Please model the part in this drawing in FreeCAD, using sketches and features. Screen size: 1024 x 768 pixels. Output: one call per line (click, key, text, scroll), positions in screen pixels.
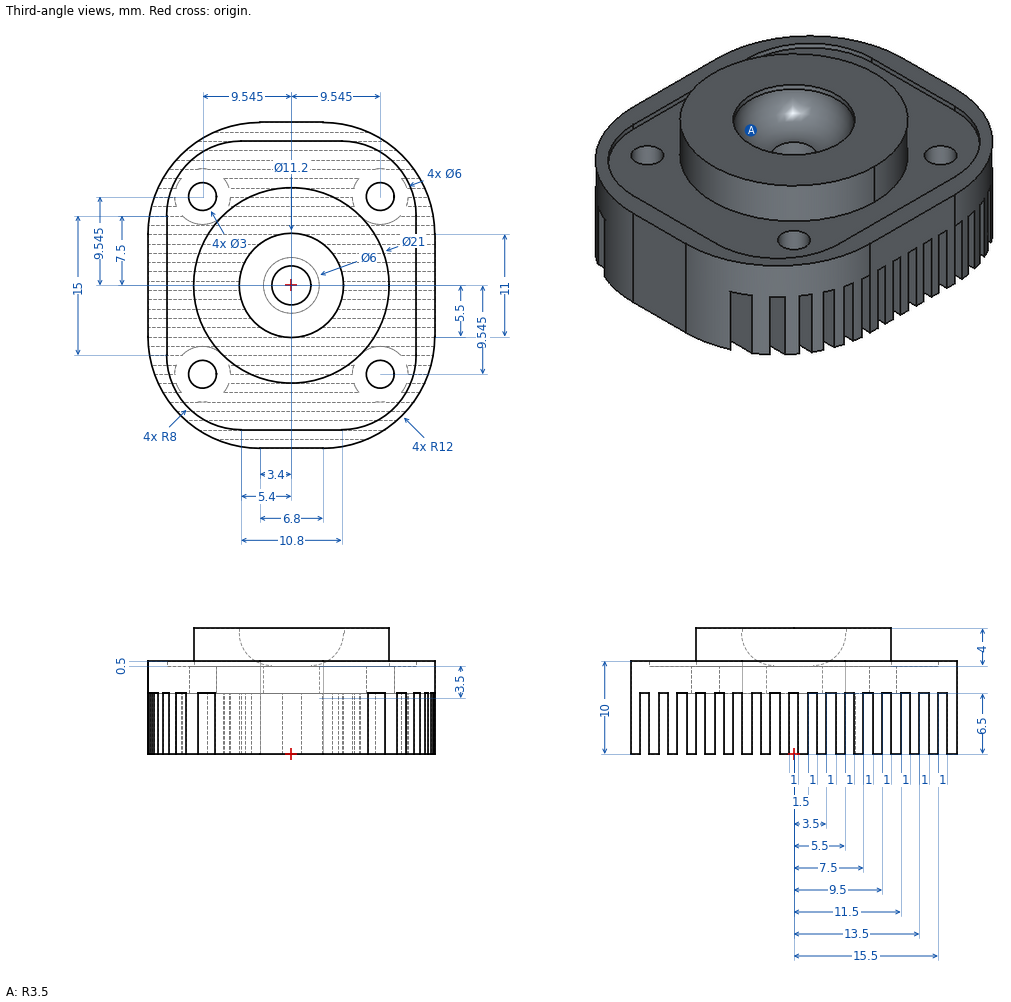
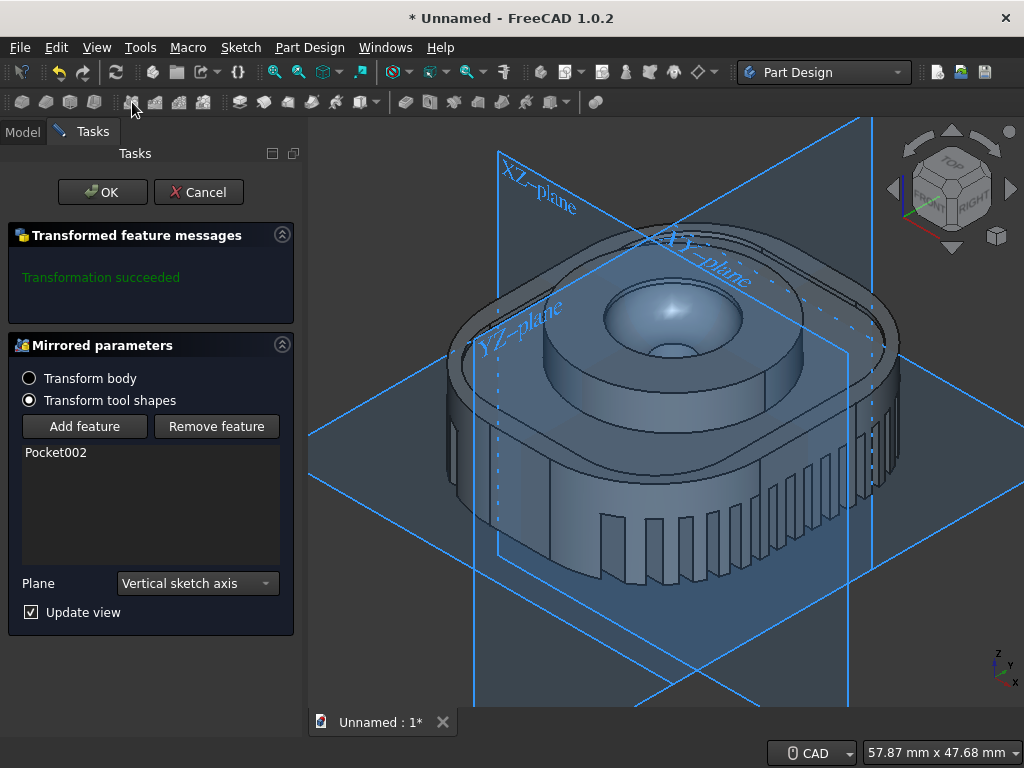
click(198, 584)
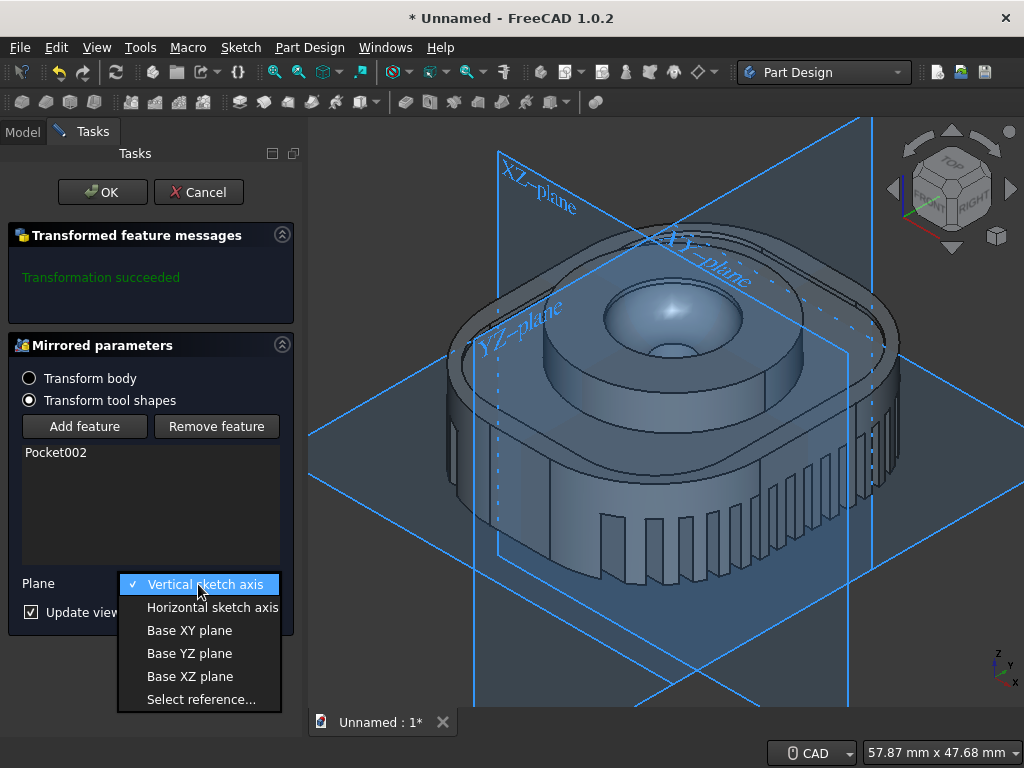
click(198, 676)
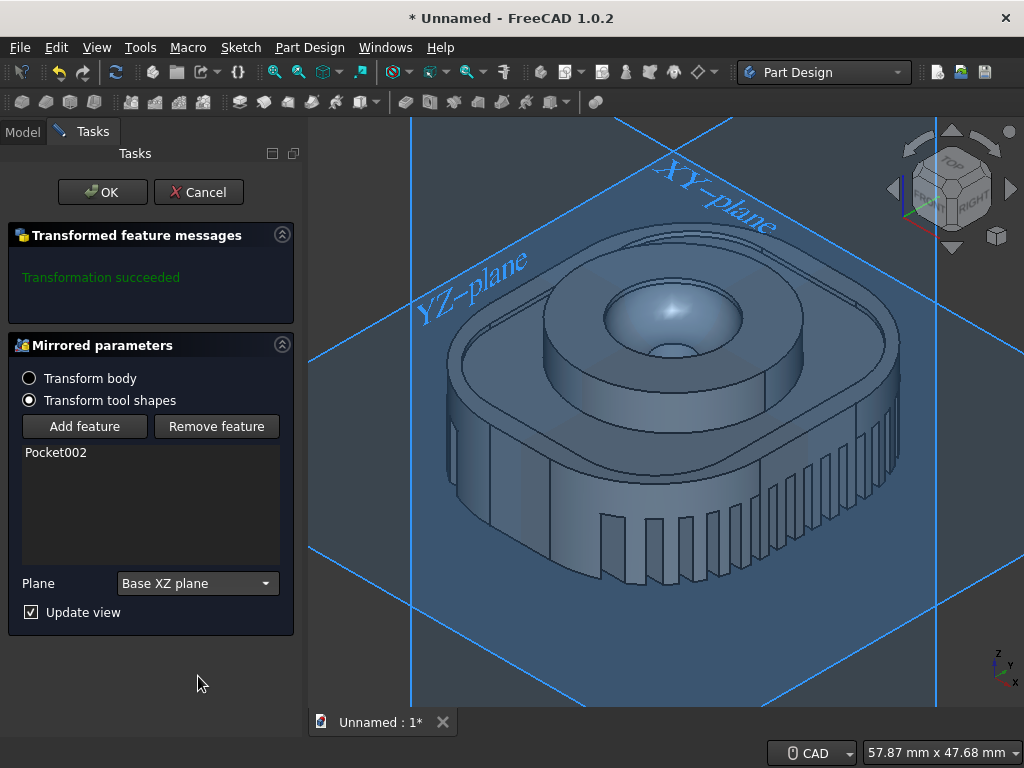
click(103, 192)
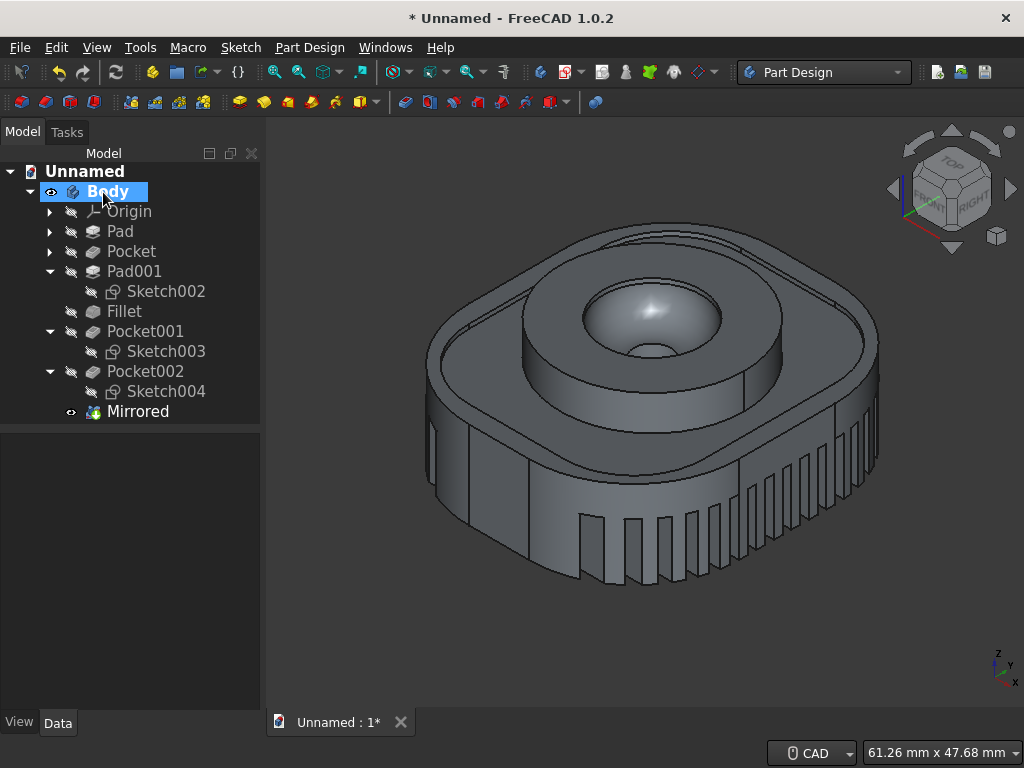
click(802, 310)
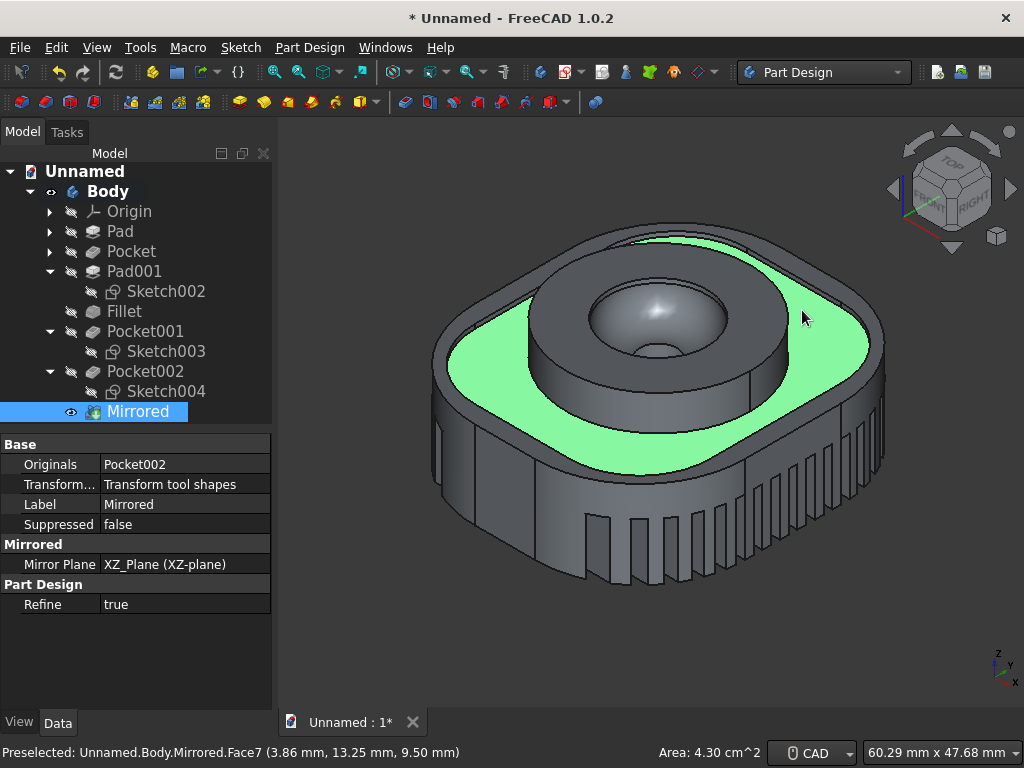
click(566, 72)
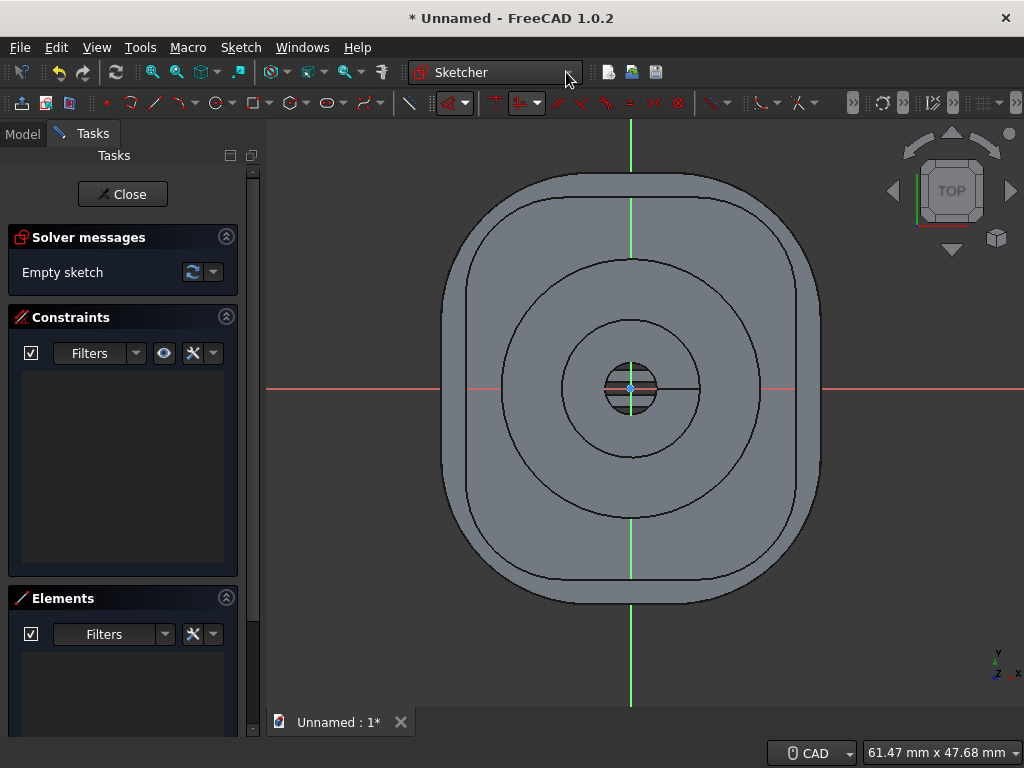
click(70, 104)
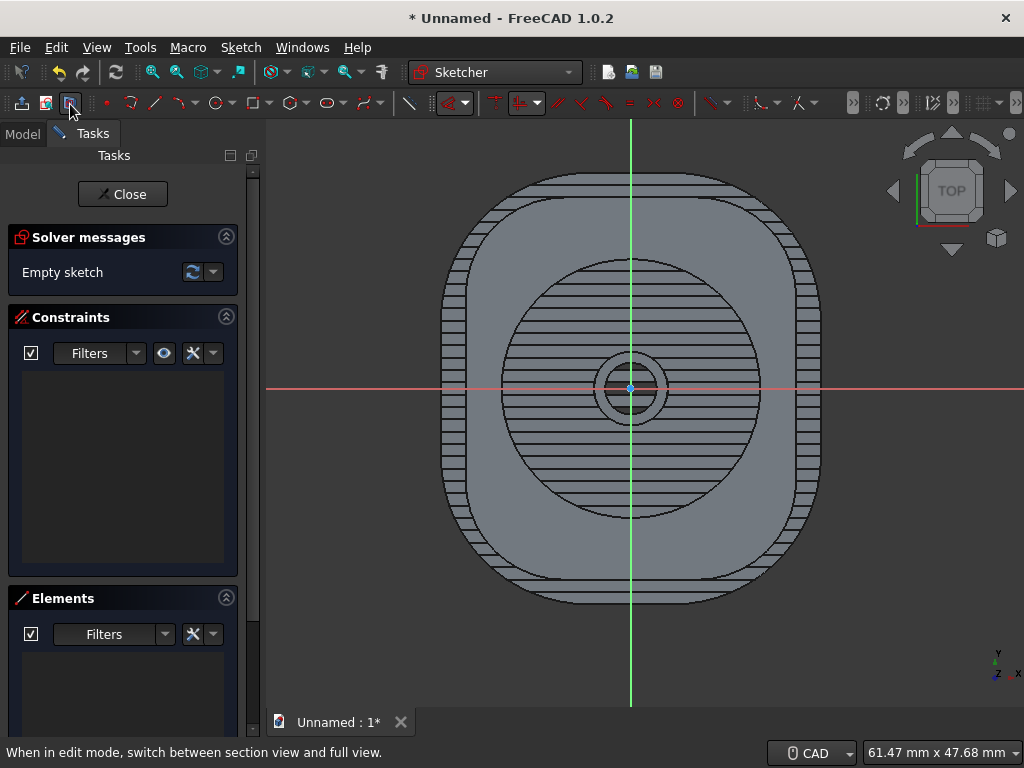
scroll(742, 339, up, 2)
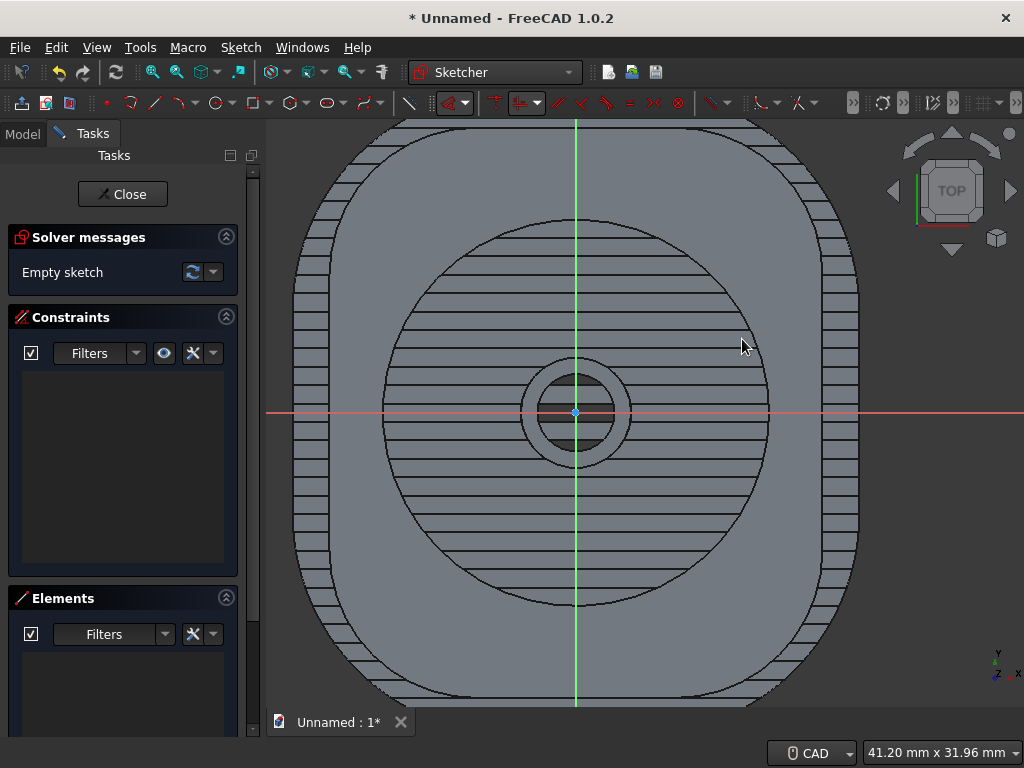
click(216, 104)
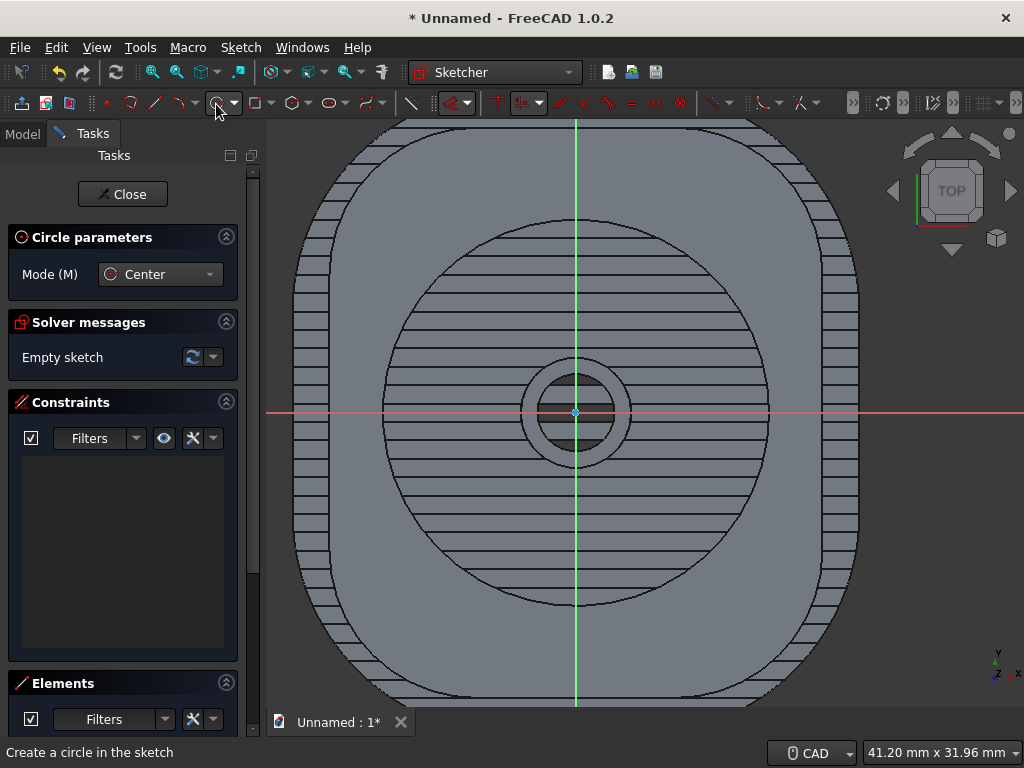
click(400, 237)
move(420, 218)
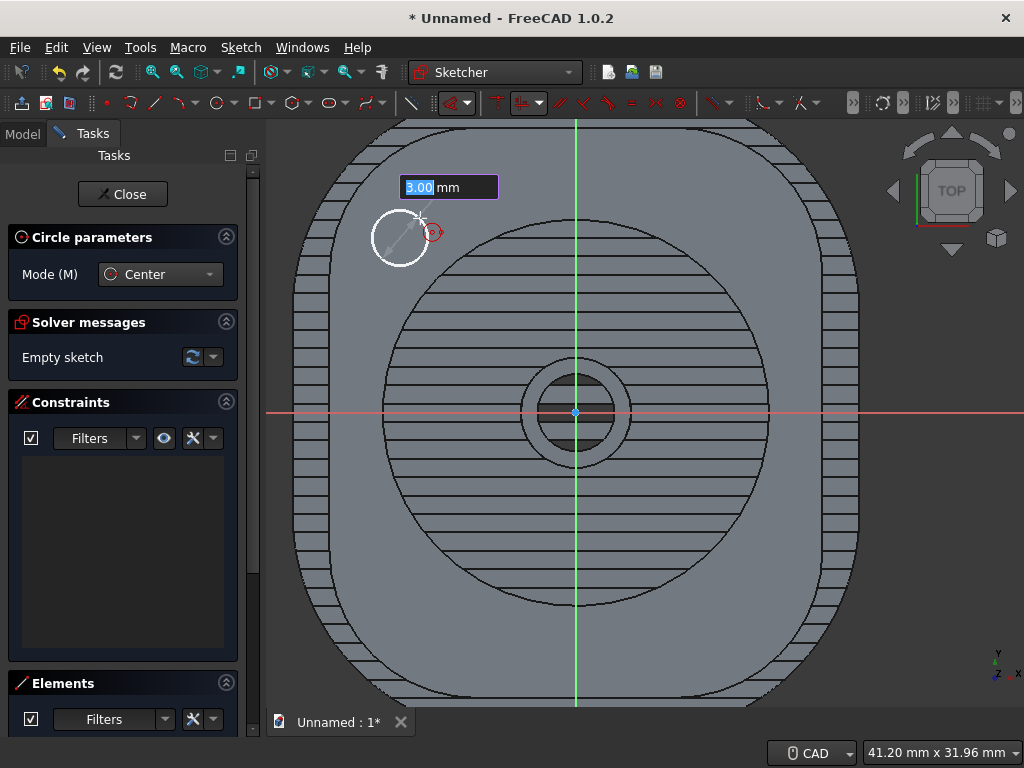
text(3)
key(Return)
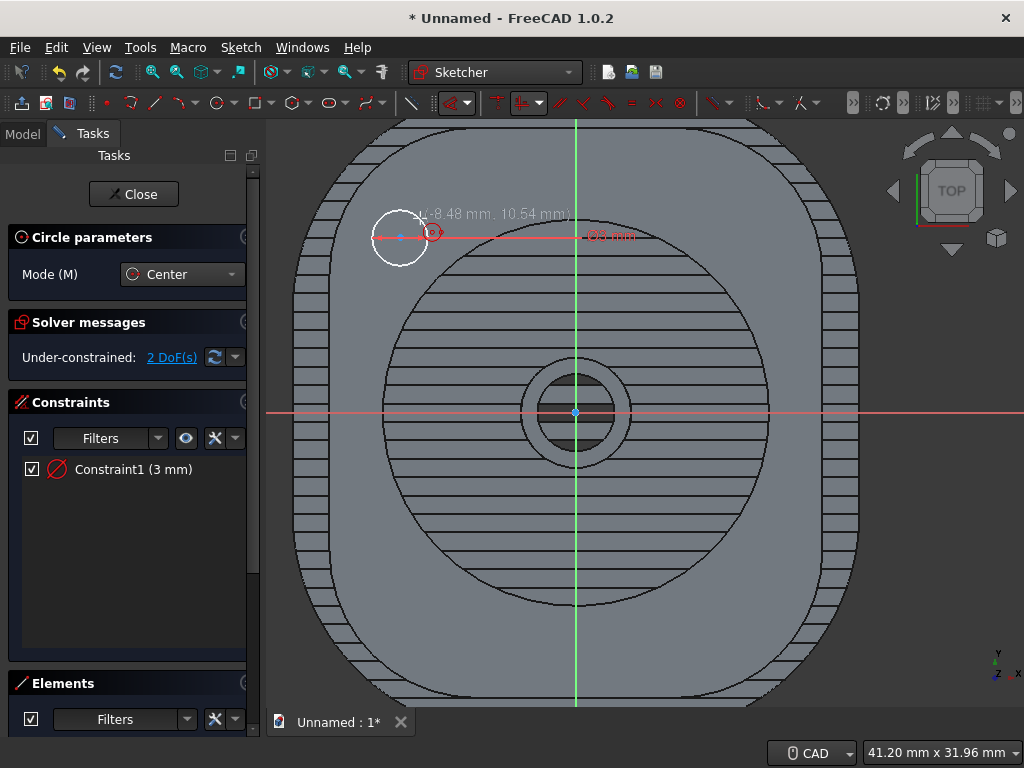
click(752, 237)
move(771, 218)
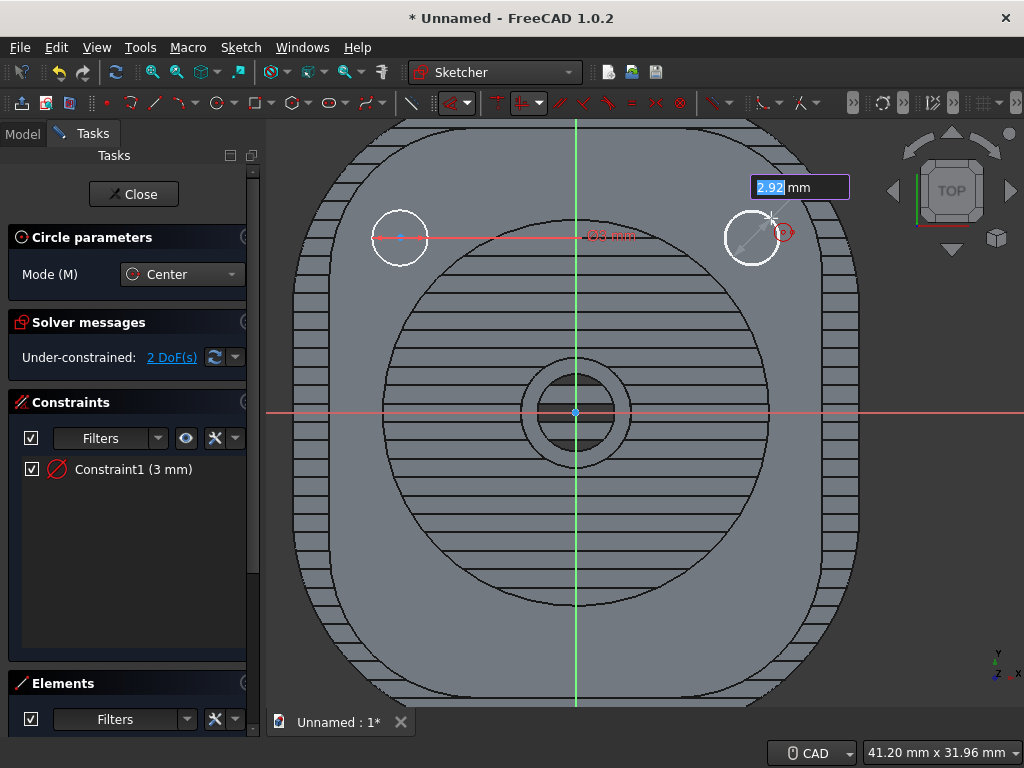
text(3)
key(Return)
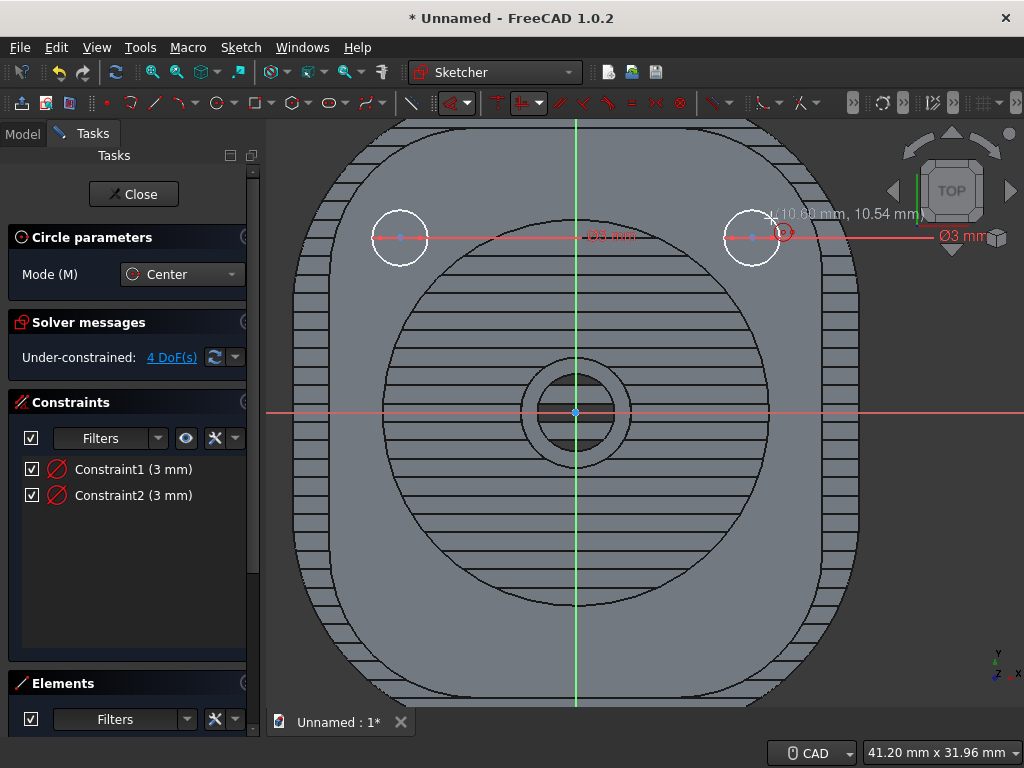
click(752, 588)
move(771, 569)